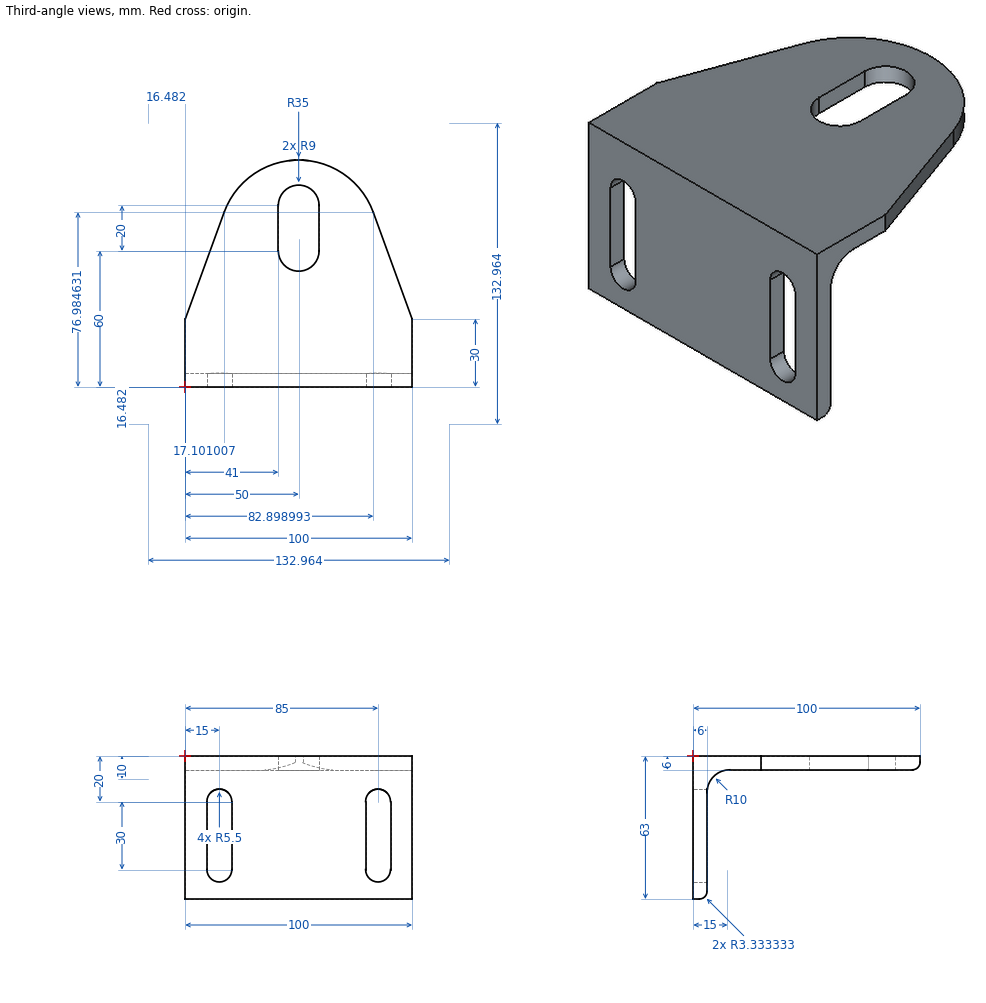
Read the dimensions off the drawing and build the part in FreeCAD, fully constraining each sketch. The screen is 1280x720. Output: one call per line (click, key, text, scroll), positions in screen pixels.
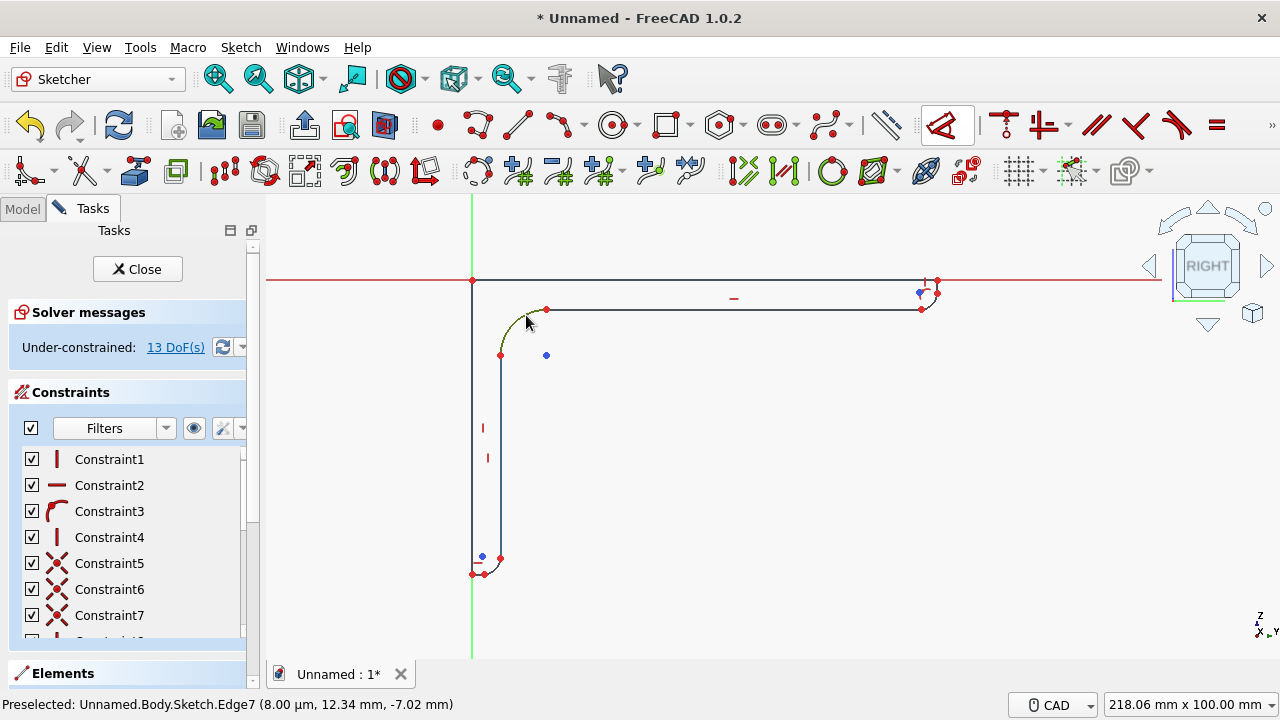
click(1178, 126)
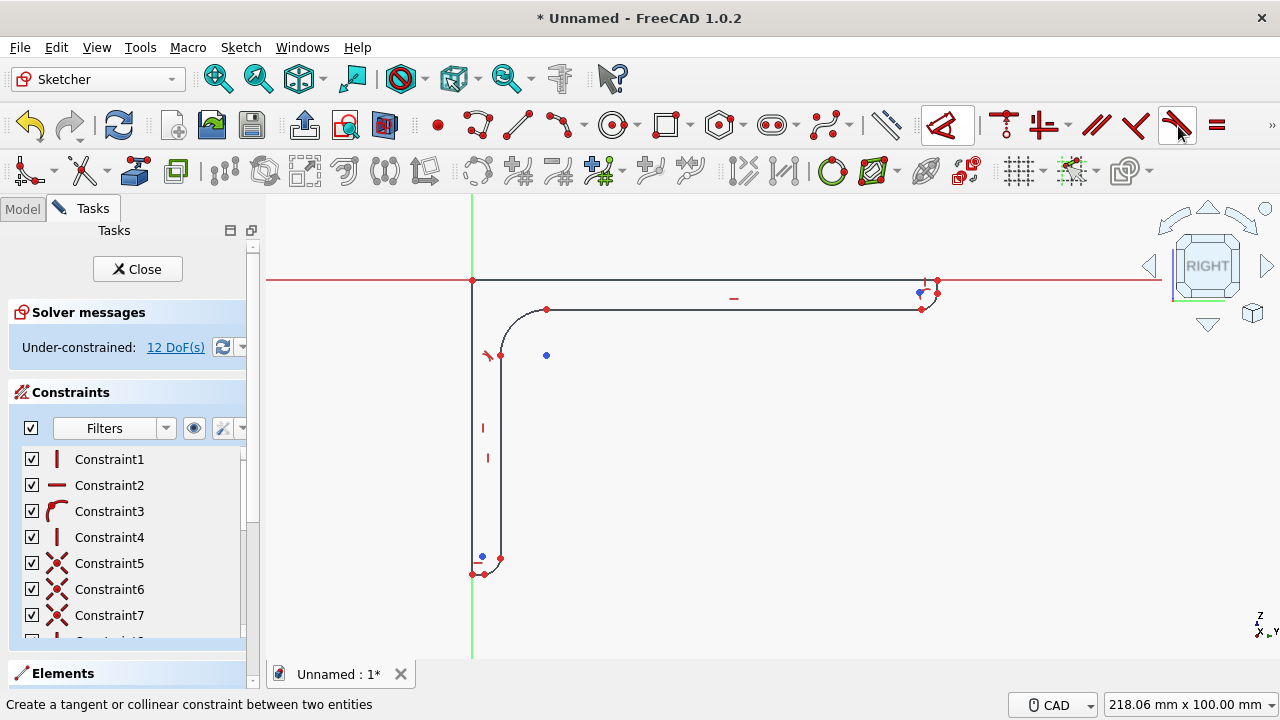
click(501, 498)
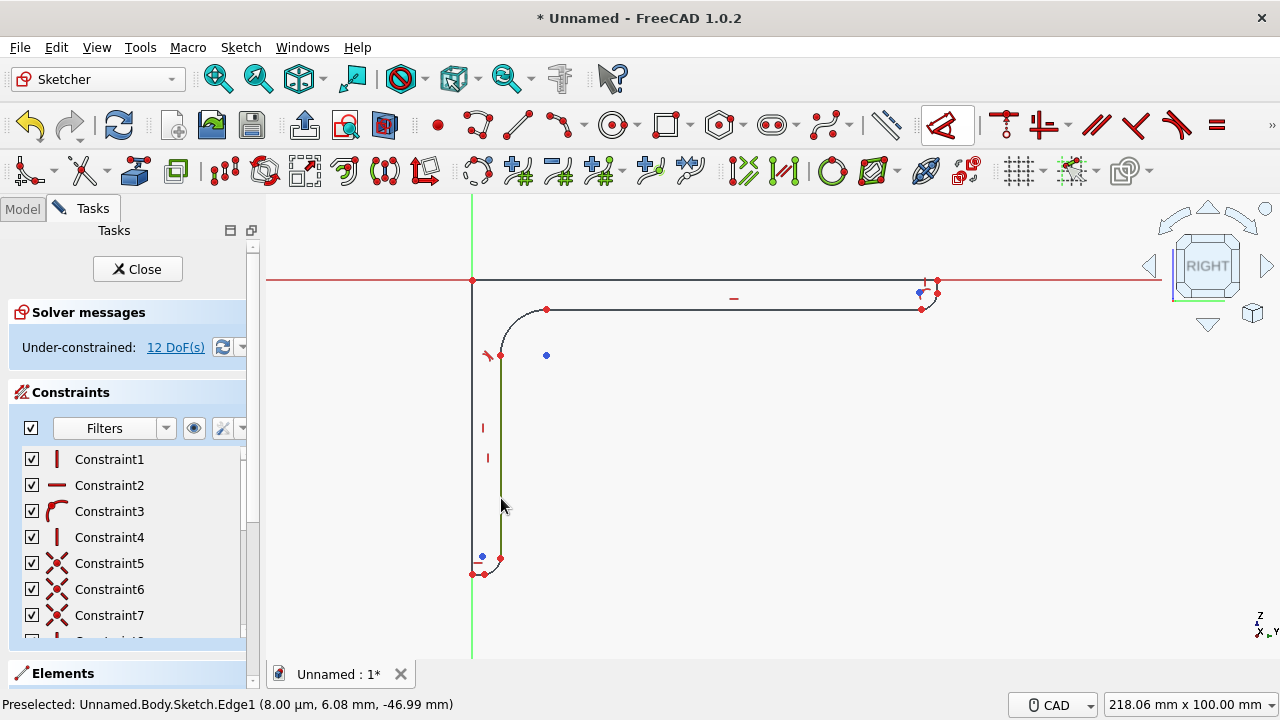
click(495, 569)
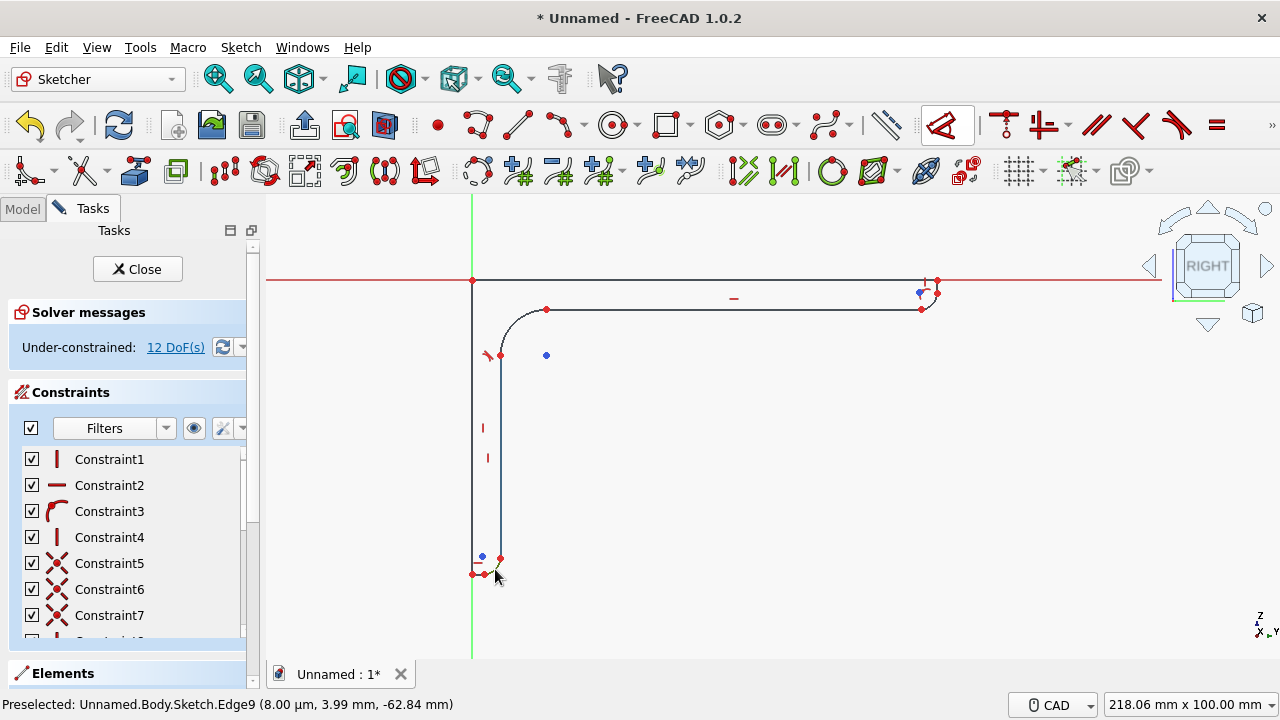
click(1178, 126)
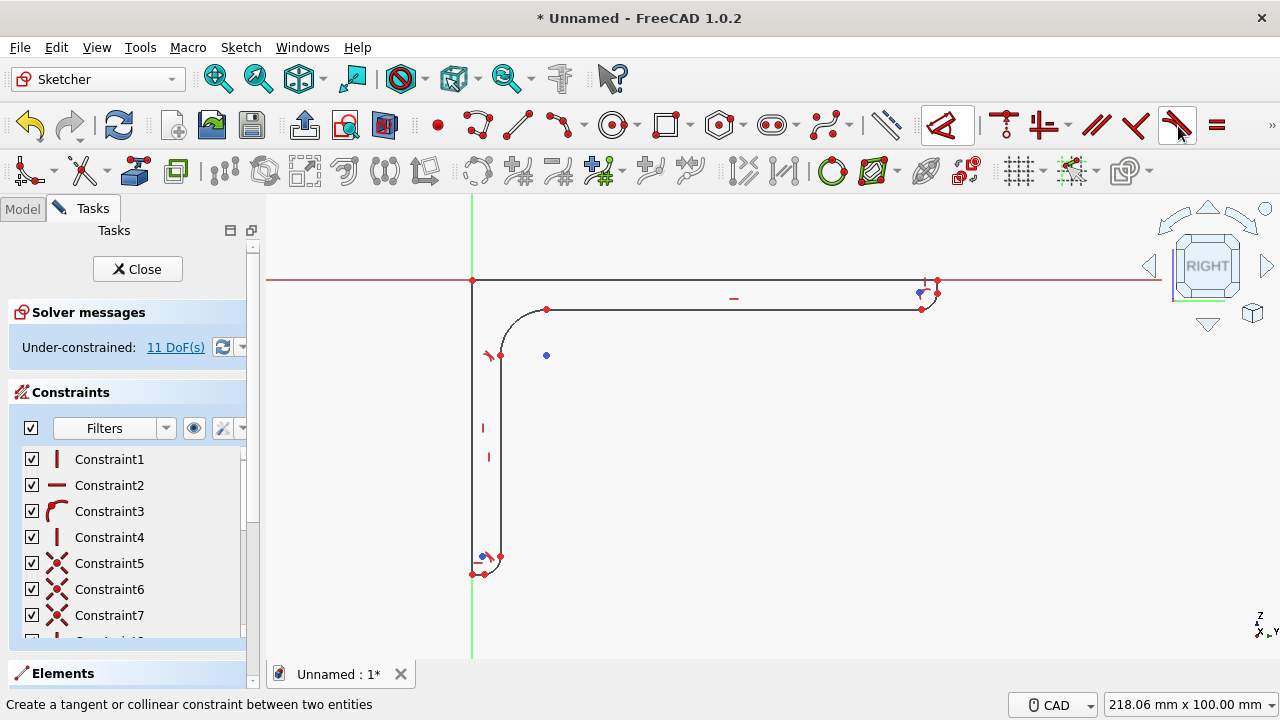
click(659, 310)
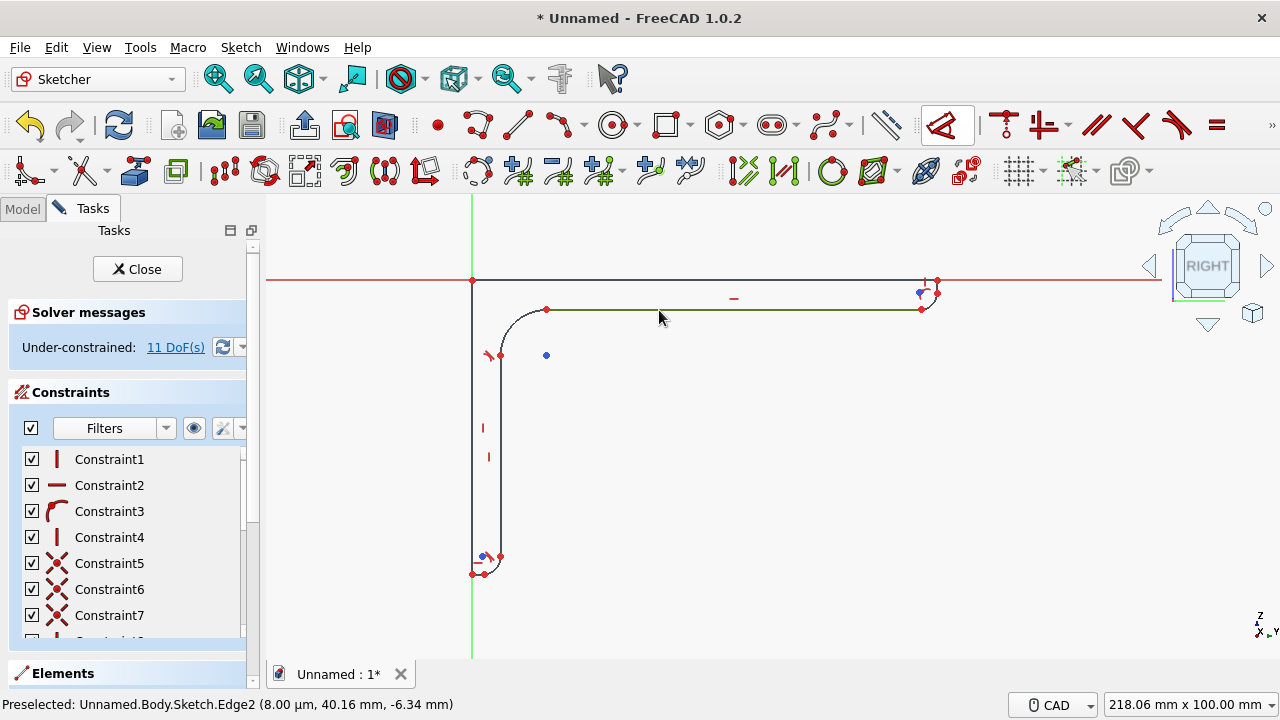
click(526, 315)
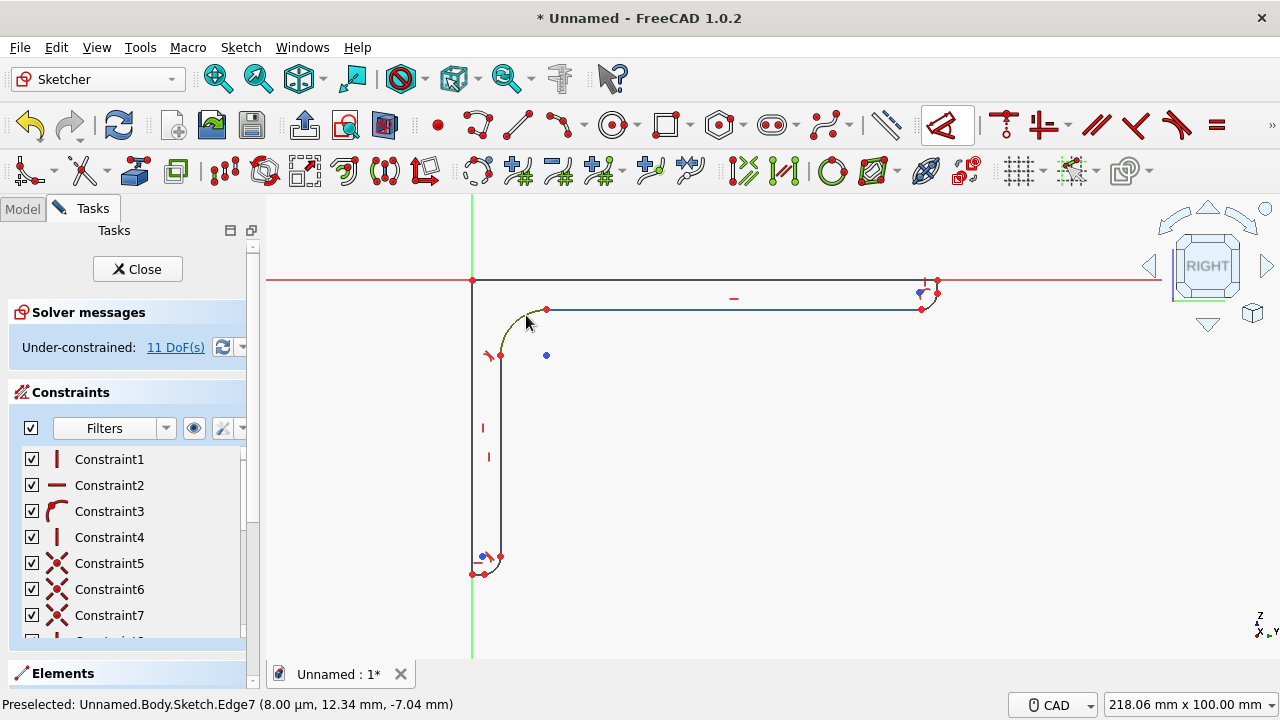
click(1178, 126)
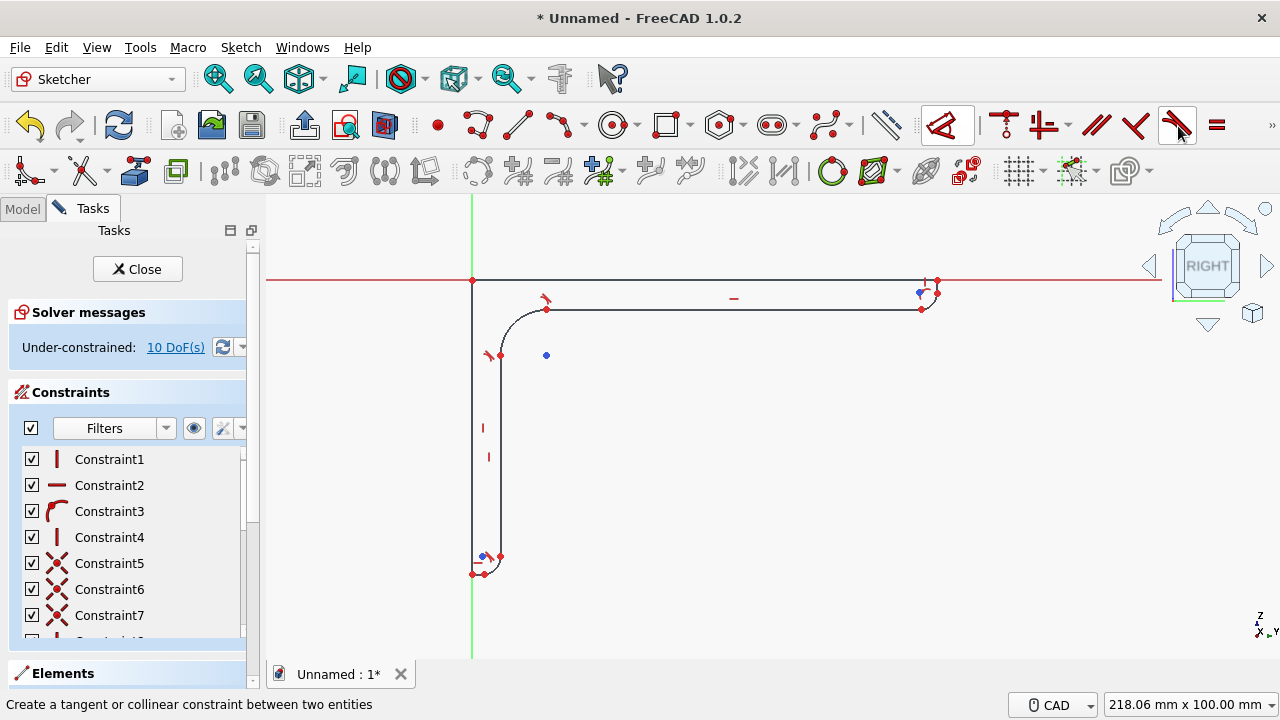
click(659, 310)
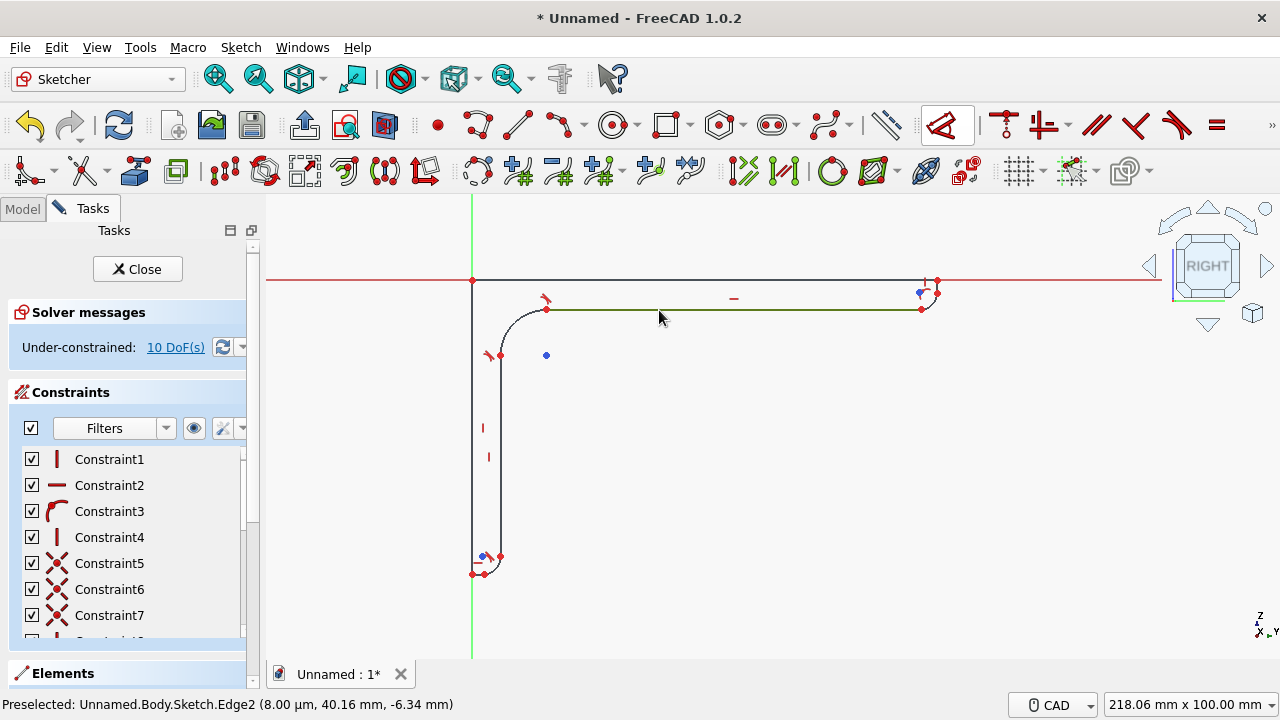
click(932, 305)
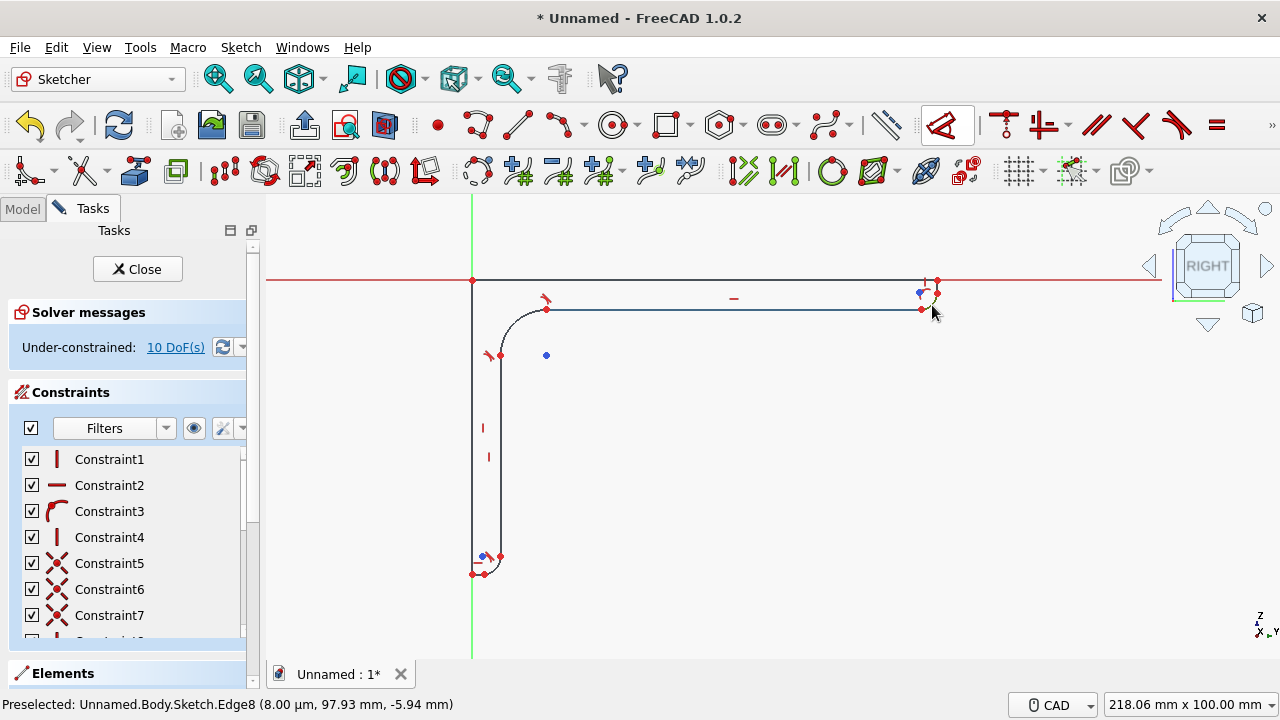
click(1178, 126)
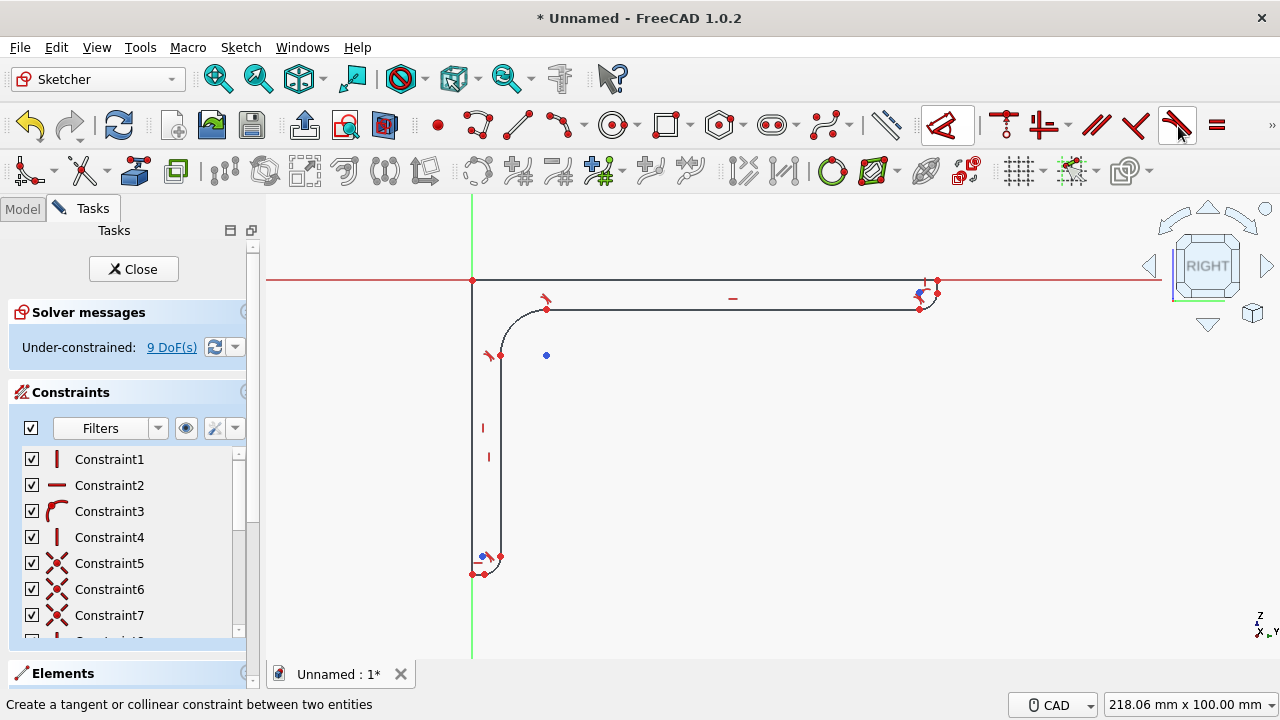
scroll(937, 287, up, 4)